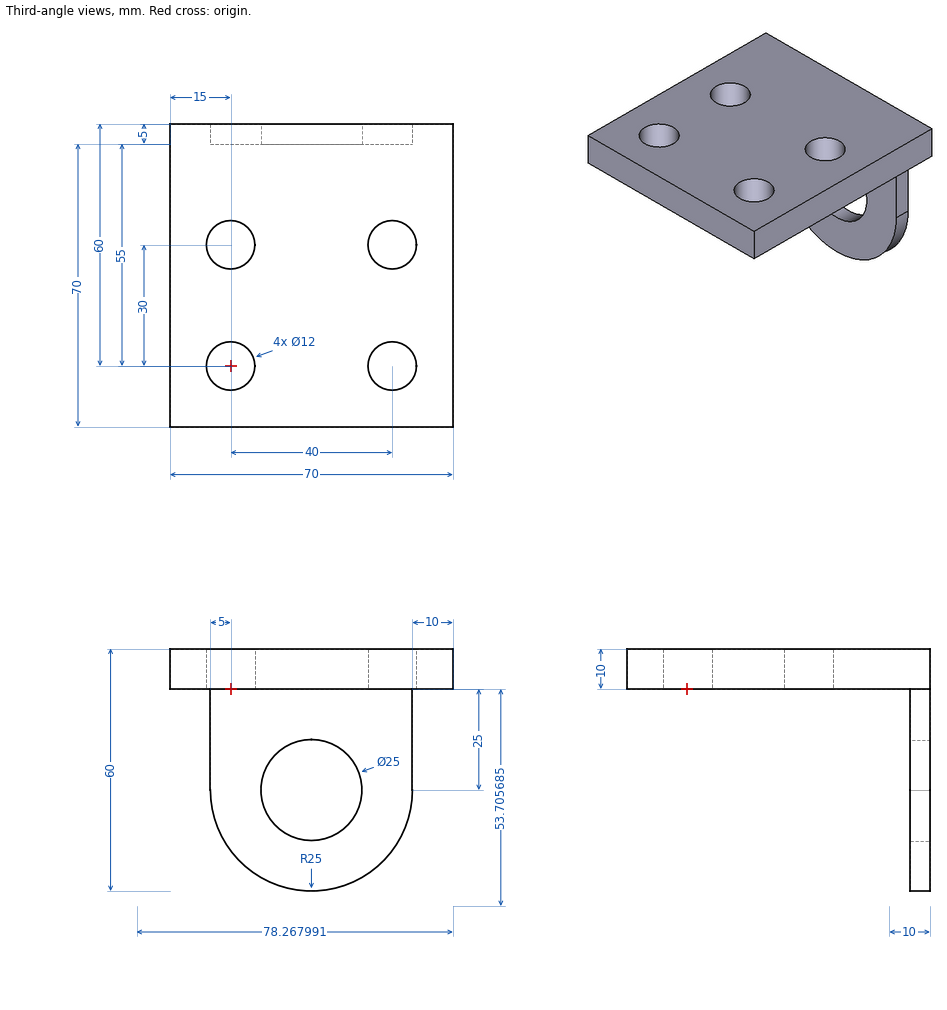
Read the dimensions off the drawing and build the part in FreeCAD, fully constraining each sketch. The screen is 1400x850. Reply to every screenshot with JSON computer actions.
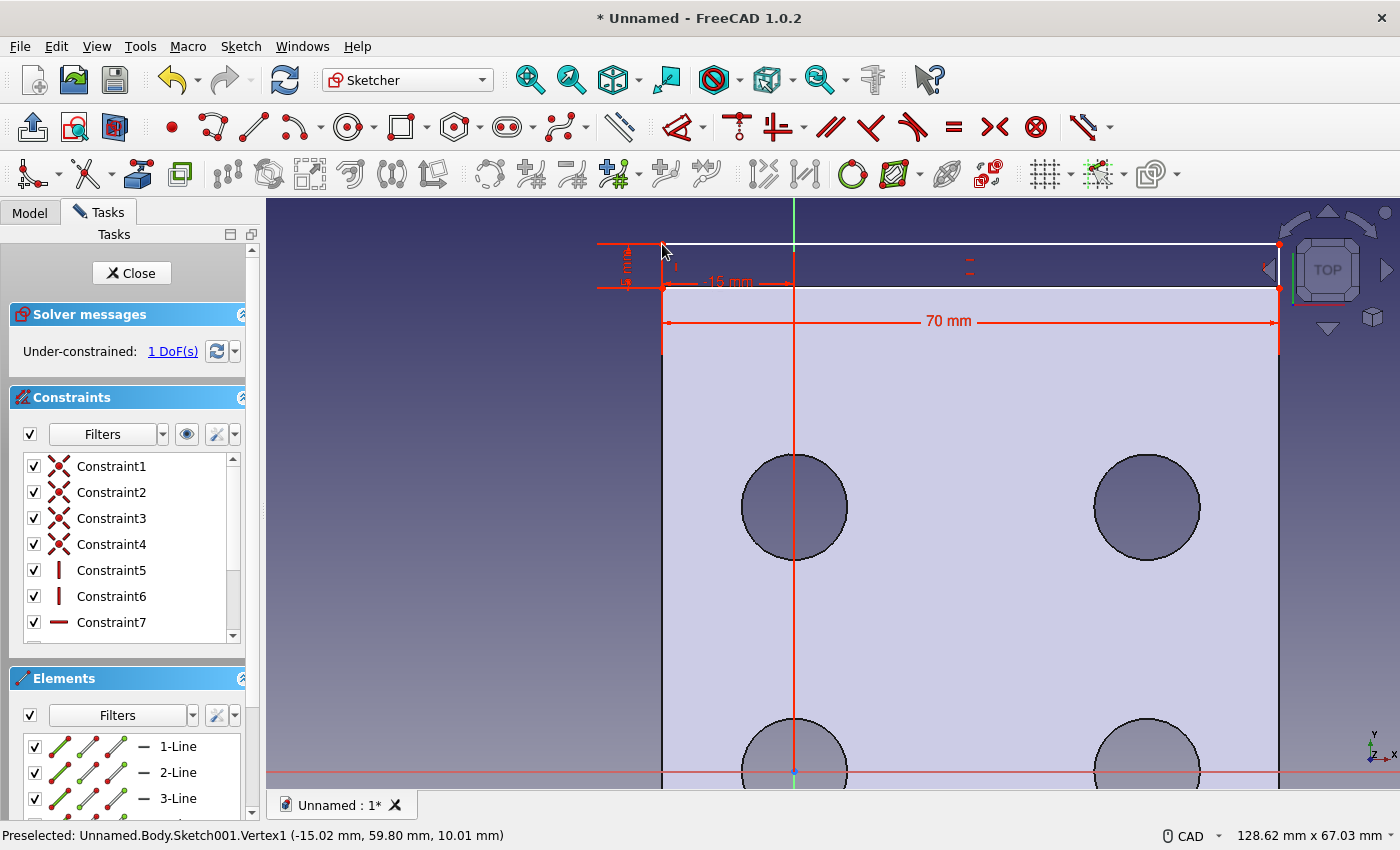
{"action": "left_click", "coordinate": [662, 244]}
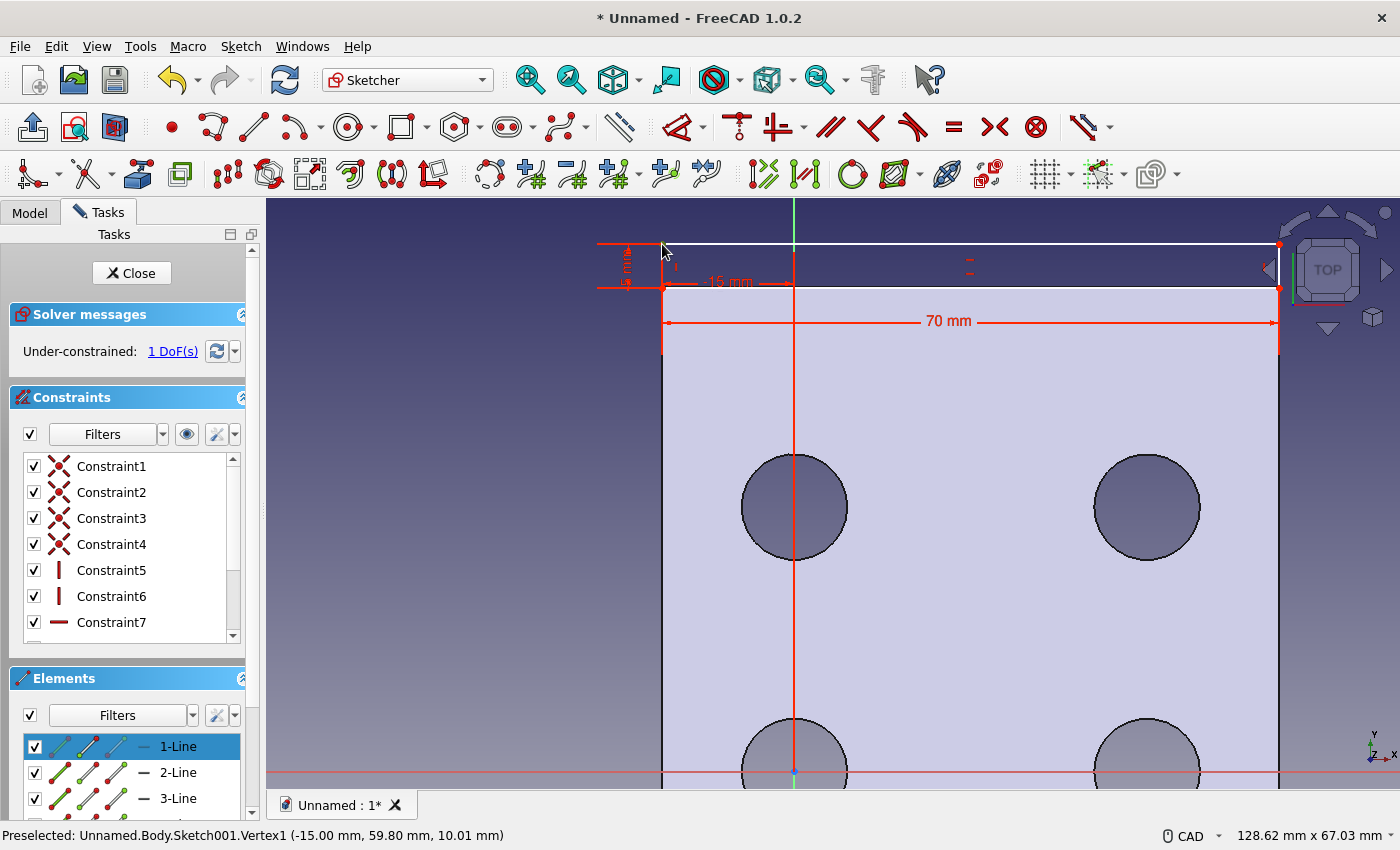
{"action": "left_click", "coordinate": [702, 128]}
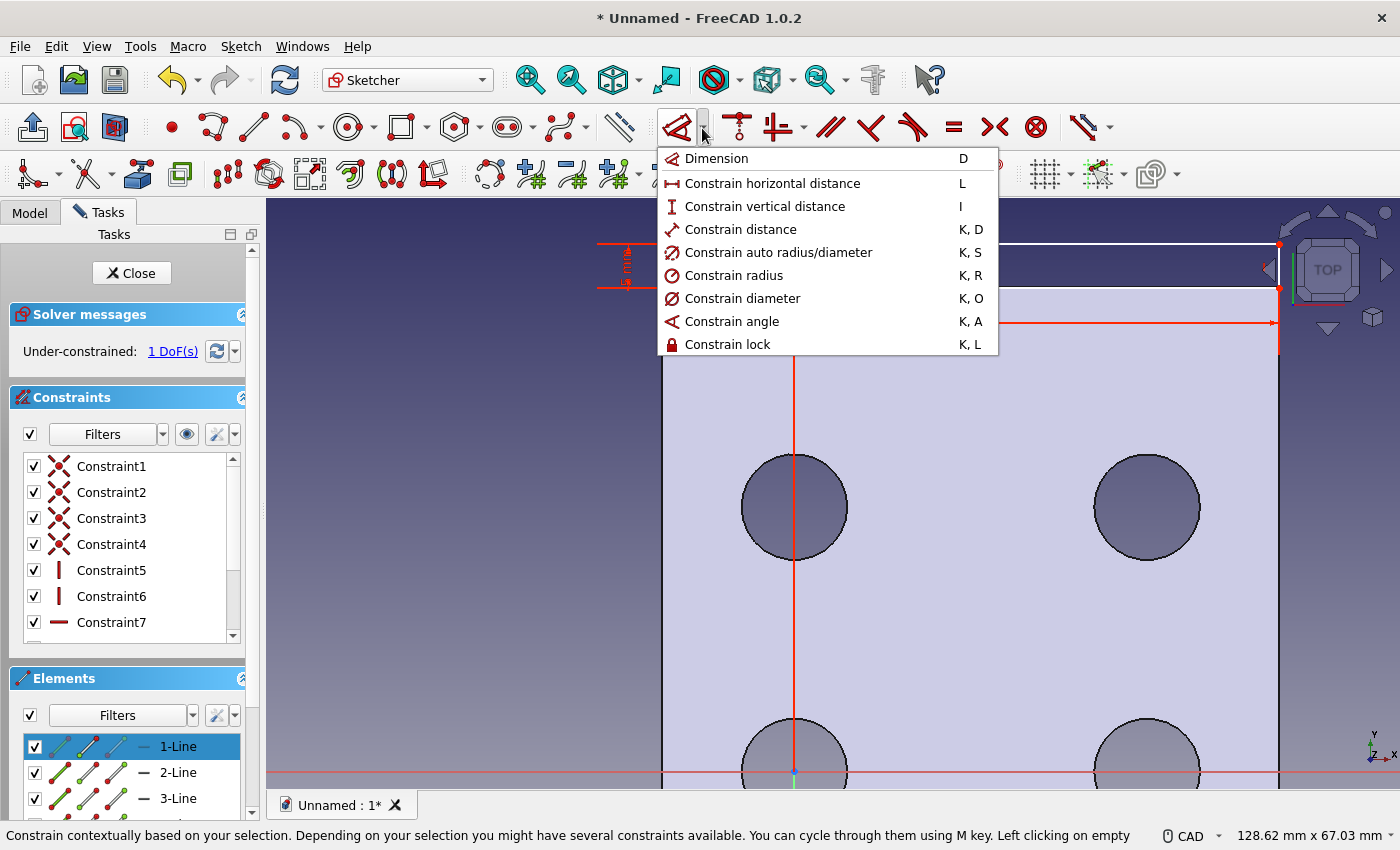
{"action": "left_click", "coordinate": [828, 206]}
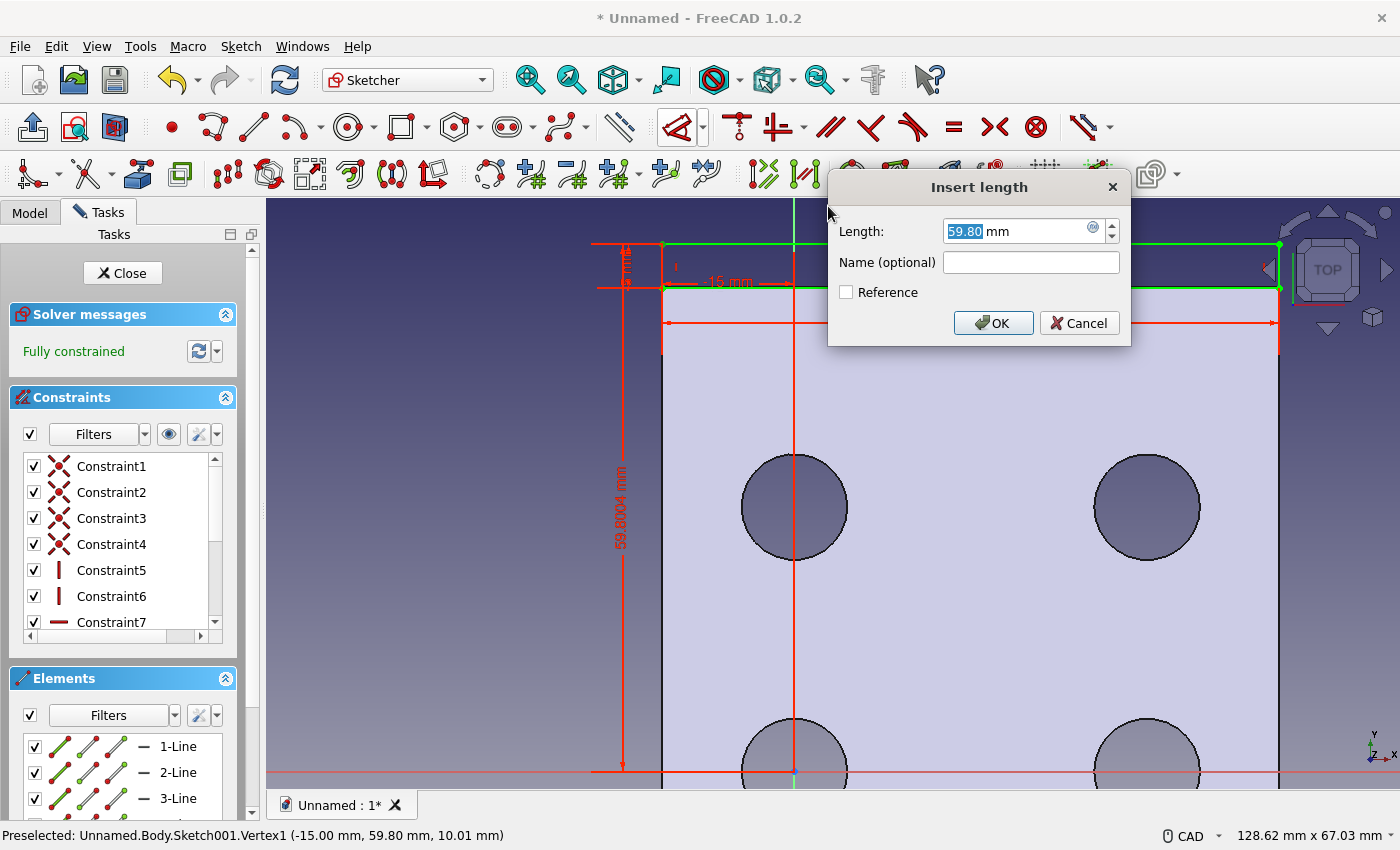
{"action": "type", "text": "60"}
{"action": "key", "text": "Return"}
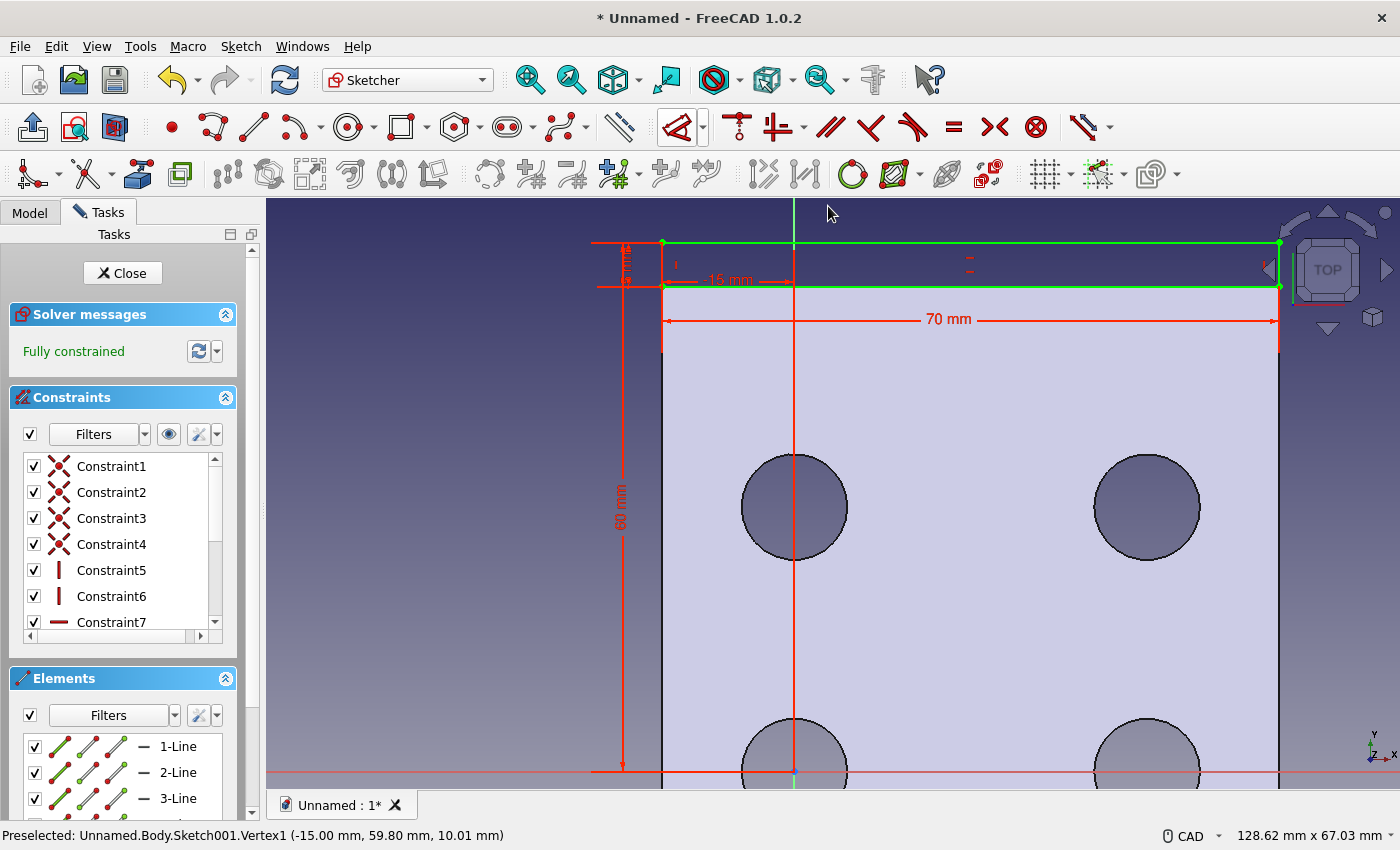
{"action": "left_click", "coordinate": [123, 273]}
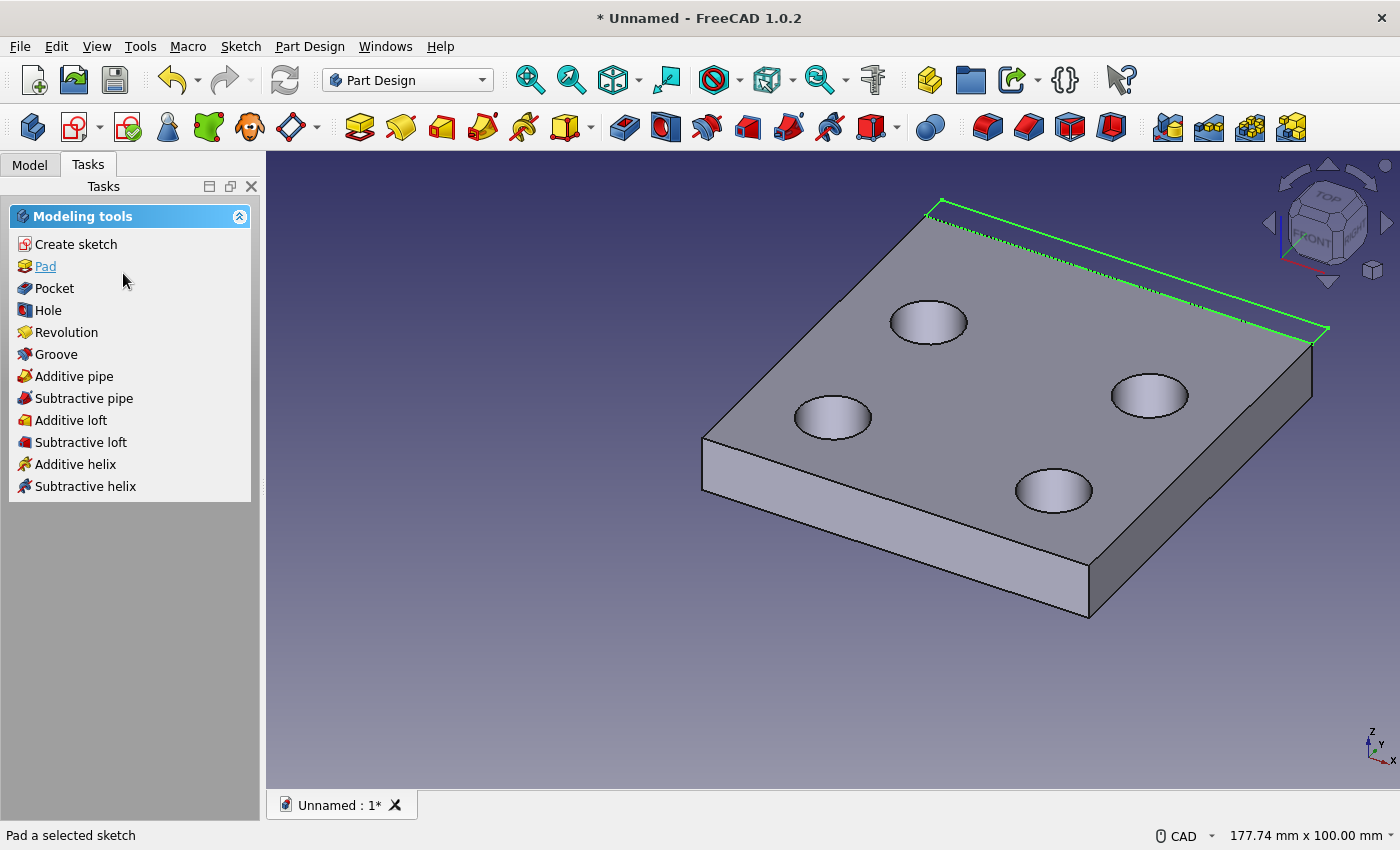
{"action": "left_click", "coordinate": [360, 128]}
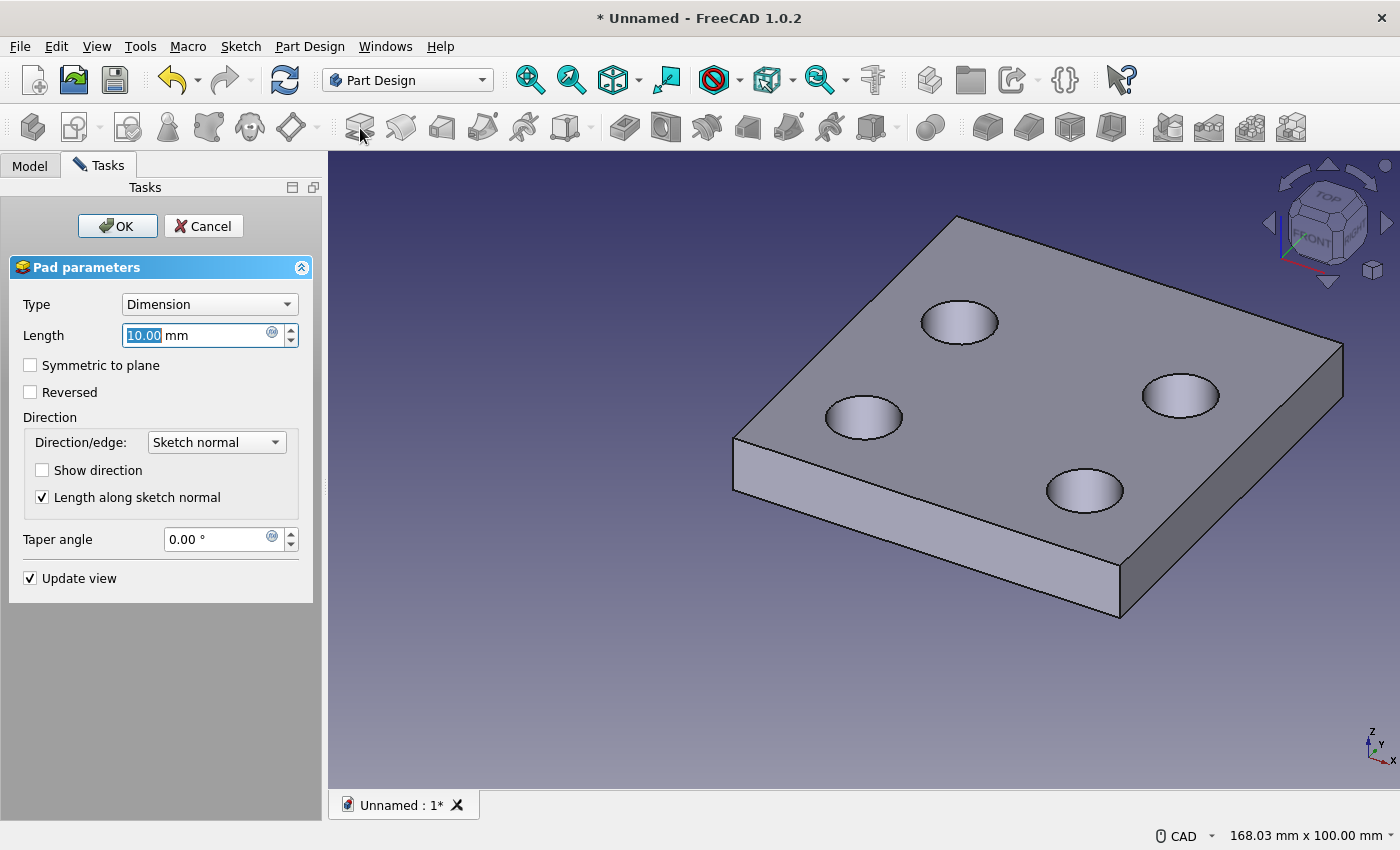
{"action": "type", "text": "60"}
{"action": "key", "text": "Tab"}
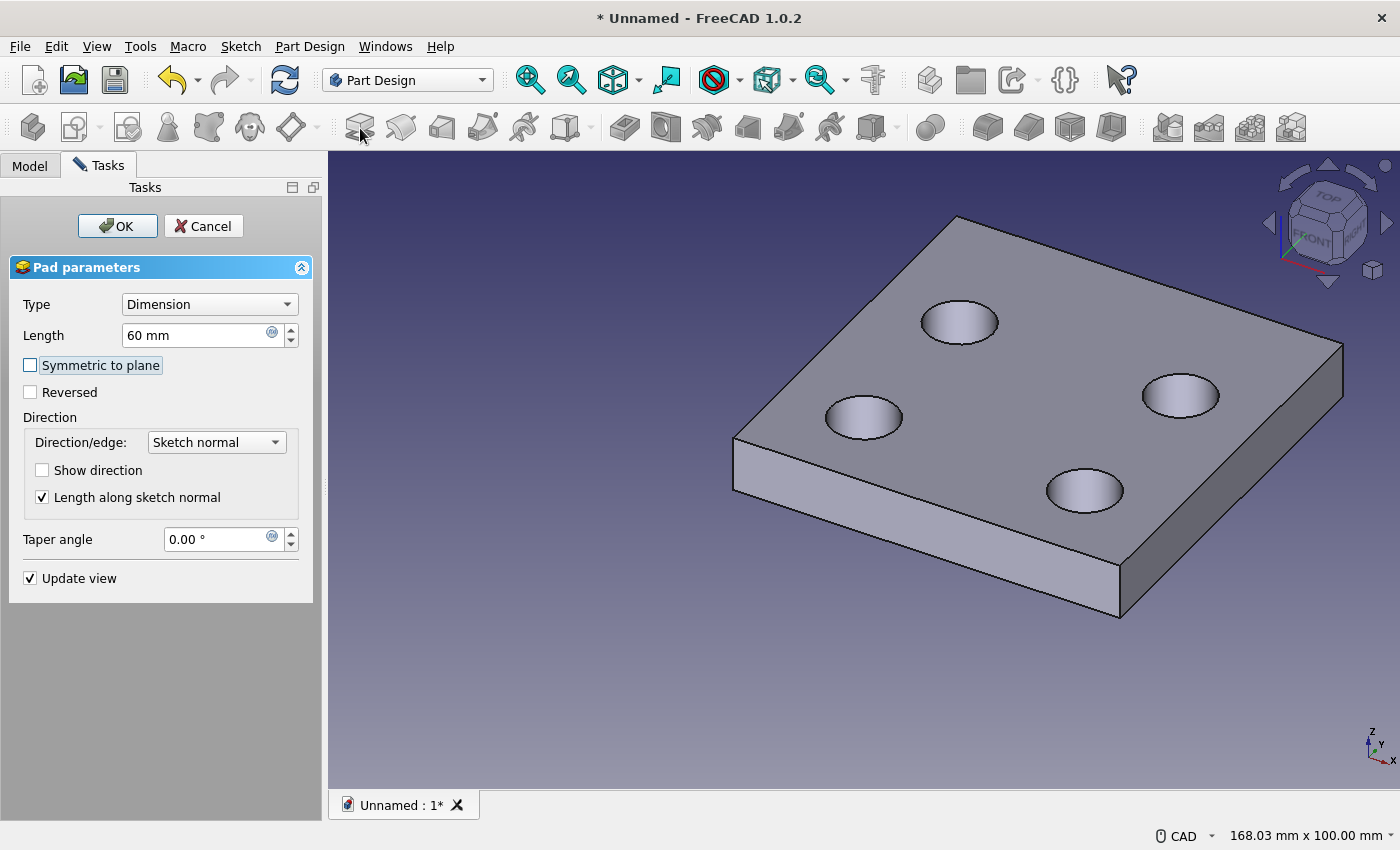
{"action": "left_click", "coordinate": [31, 392]}